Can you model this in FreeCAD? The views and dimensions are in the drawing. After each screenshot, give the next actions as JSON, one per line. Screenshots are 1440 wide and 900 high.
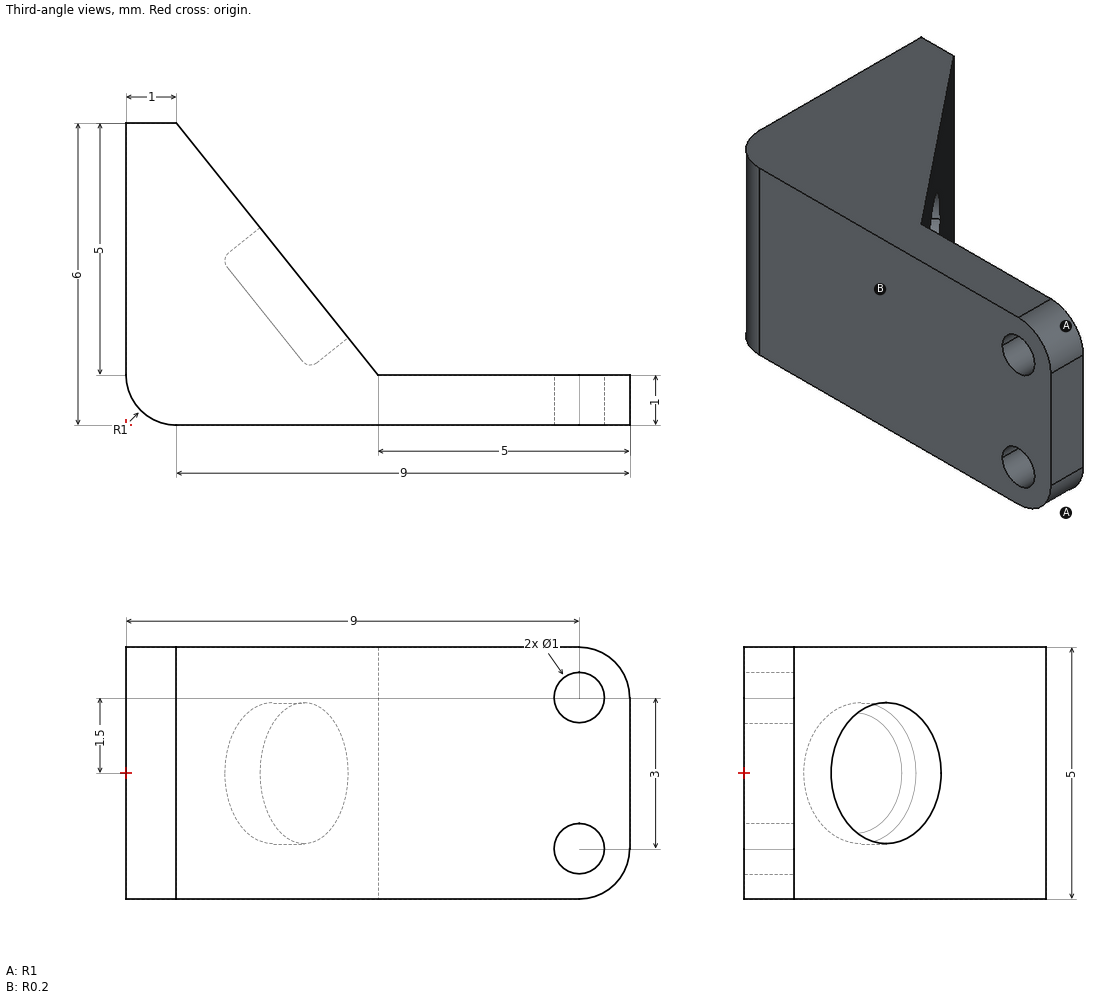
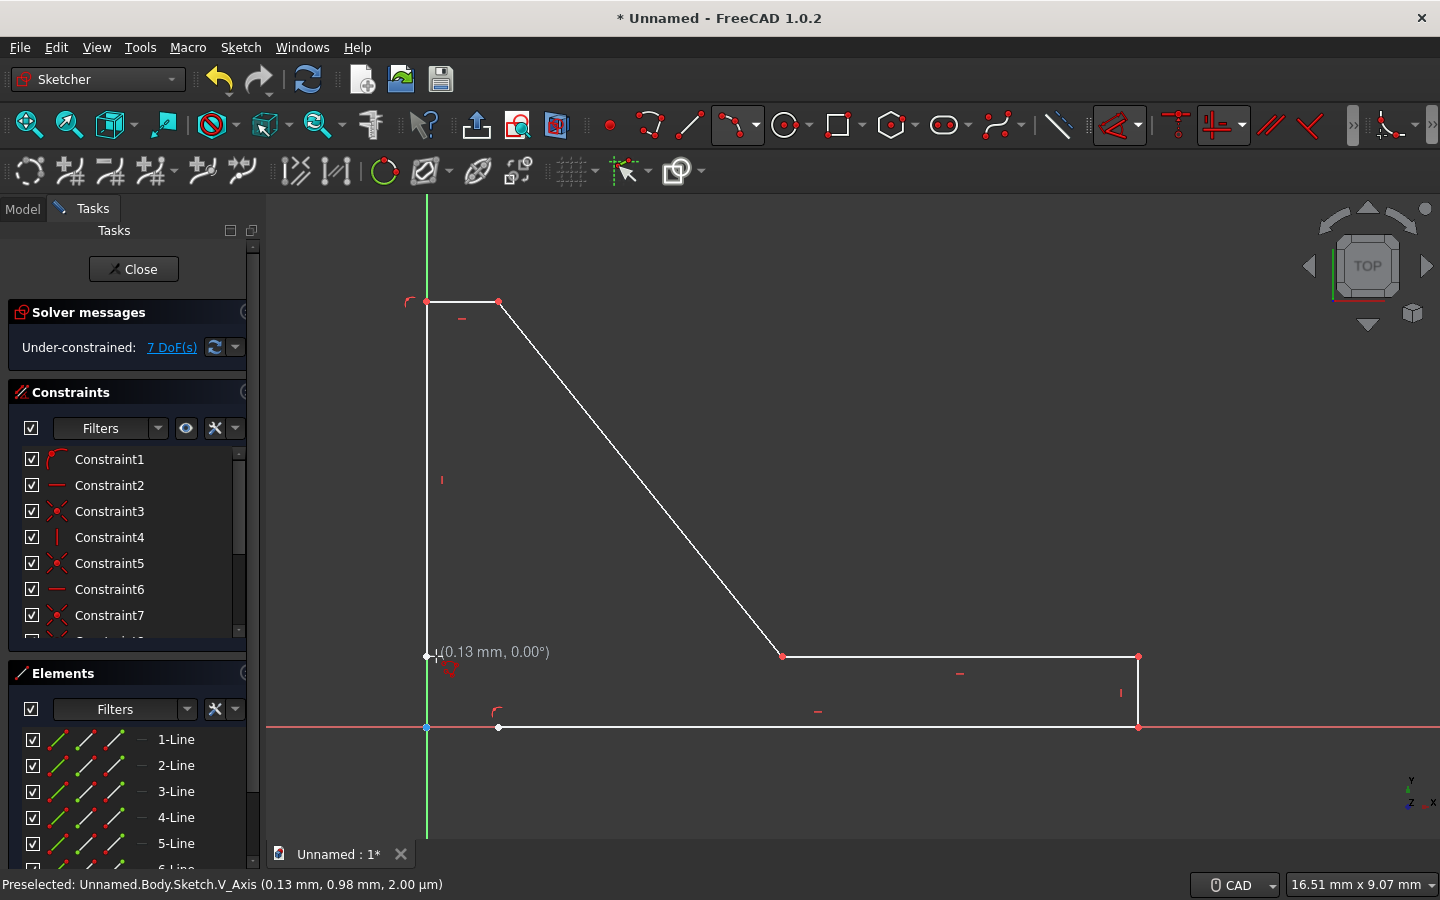
{"action": "left_click", "coordinate": [732, 126]}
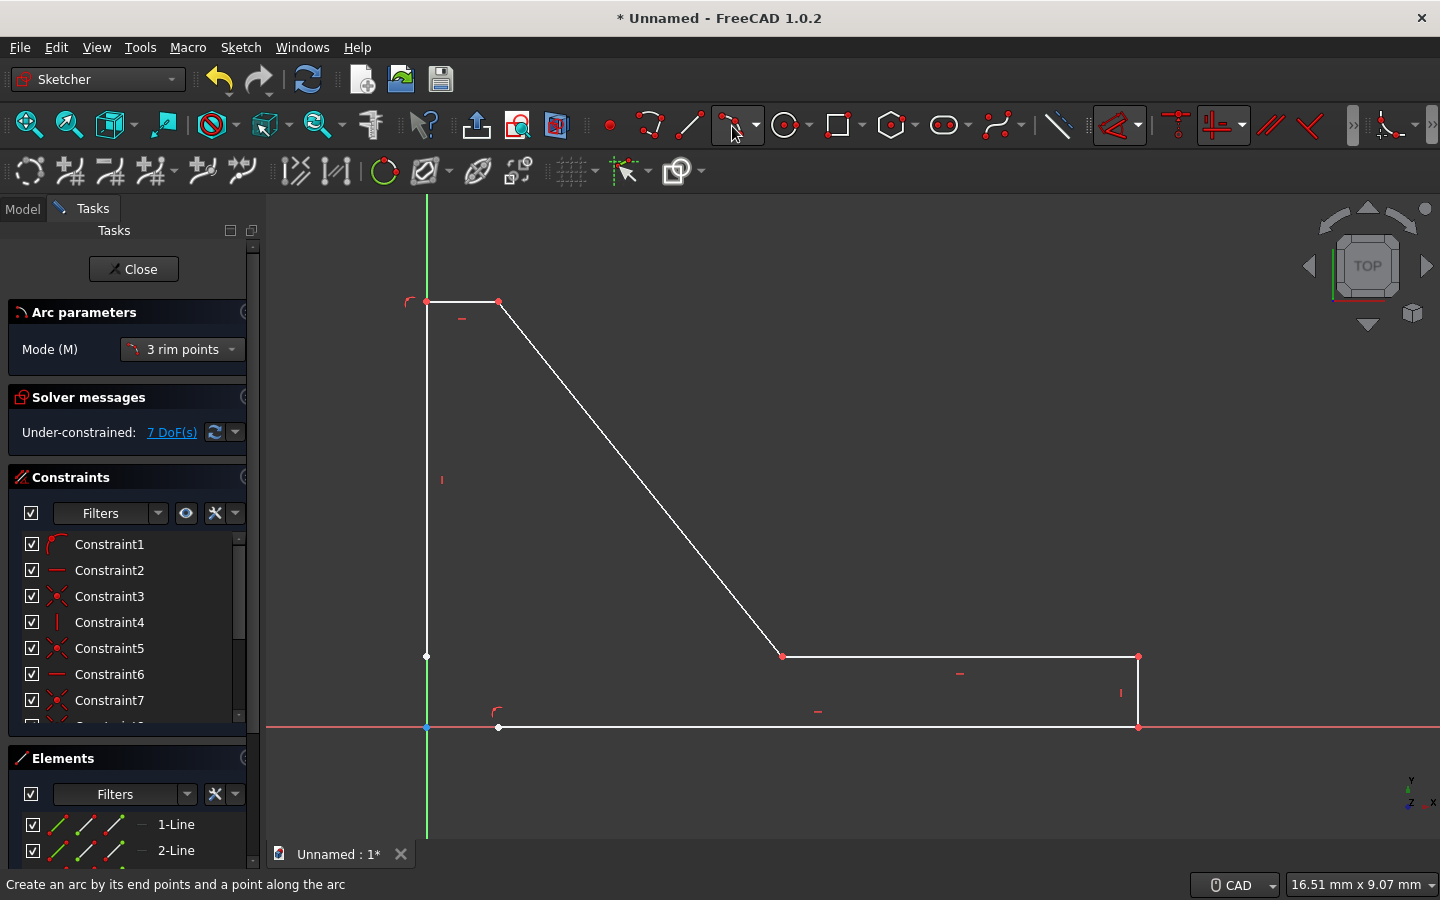
{"action": "left_click", "coordinate": [436, 656]}
{"action": "left_click", "coordinate": [498, 727]}
{"action": "left_click", "coordinate": [447, 706]}
{"action": "key", "text": "Escape"}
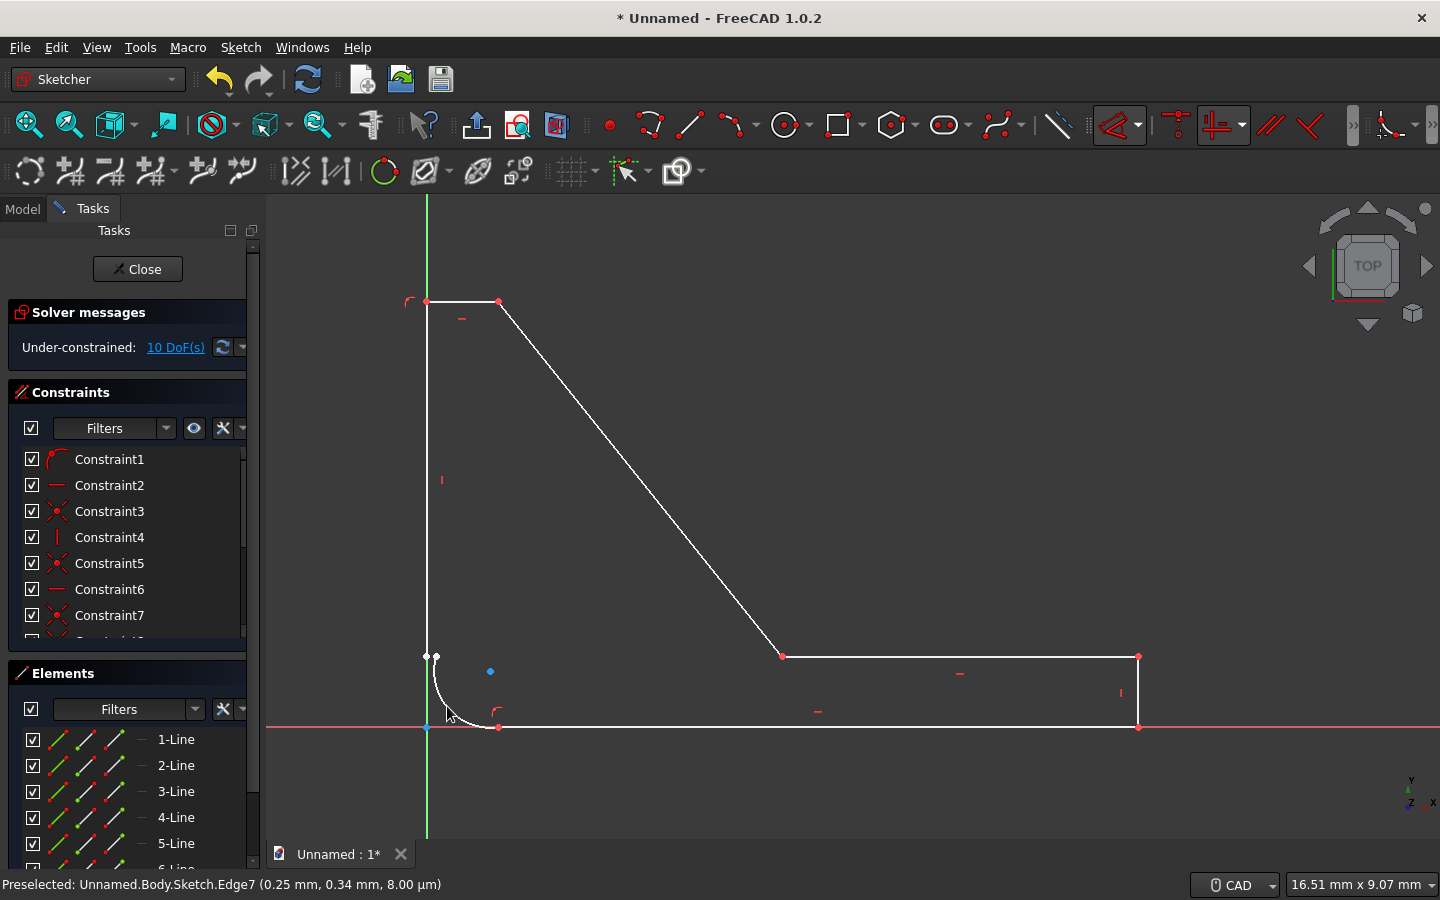
{"action": "left_click", "coordinate": [690, 727]}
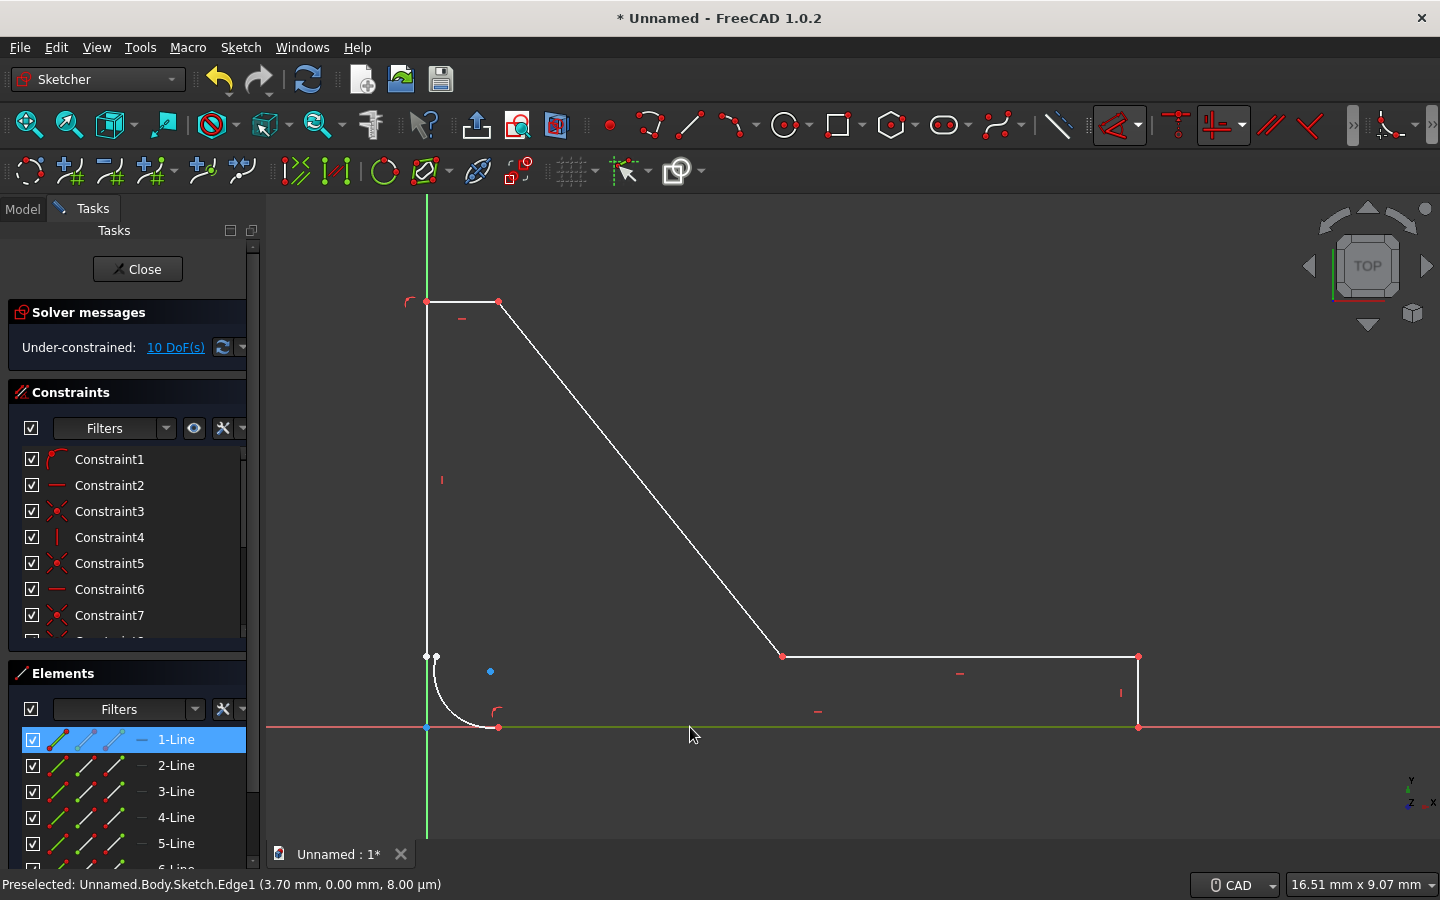
{"action": "scroll", "coordinate": [437, 690], "scroll_direction": "up", "scroll_amount": 2}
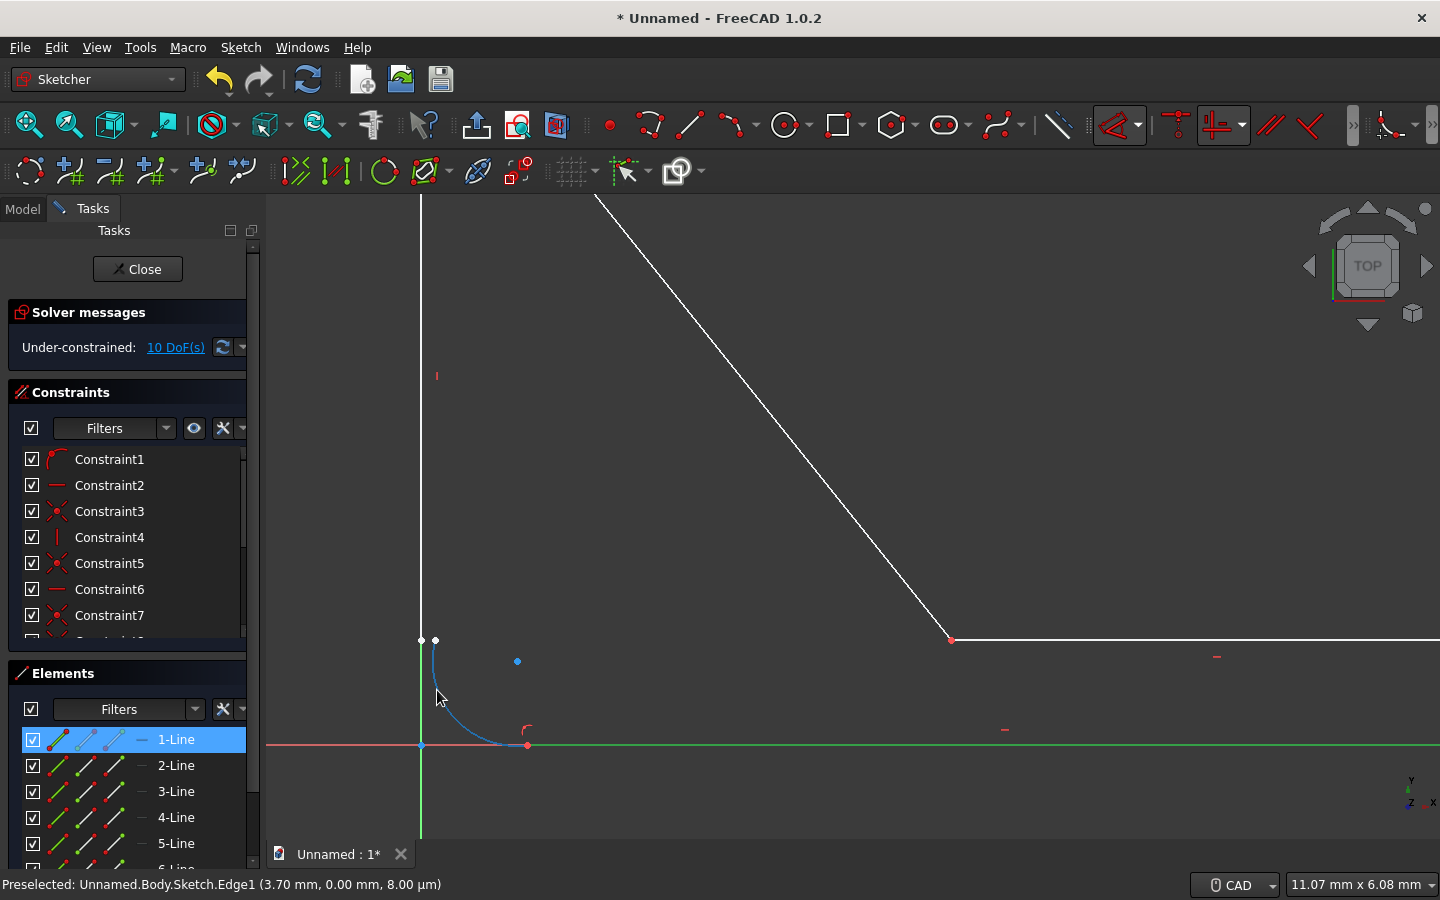
{"action": "left_click", "coordinate": [437, 689]}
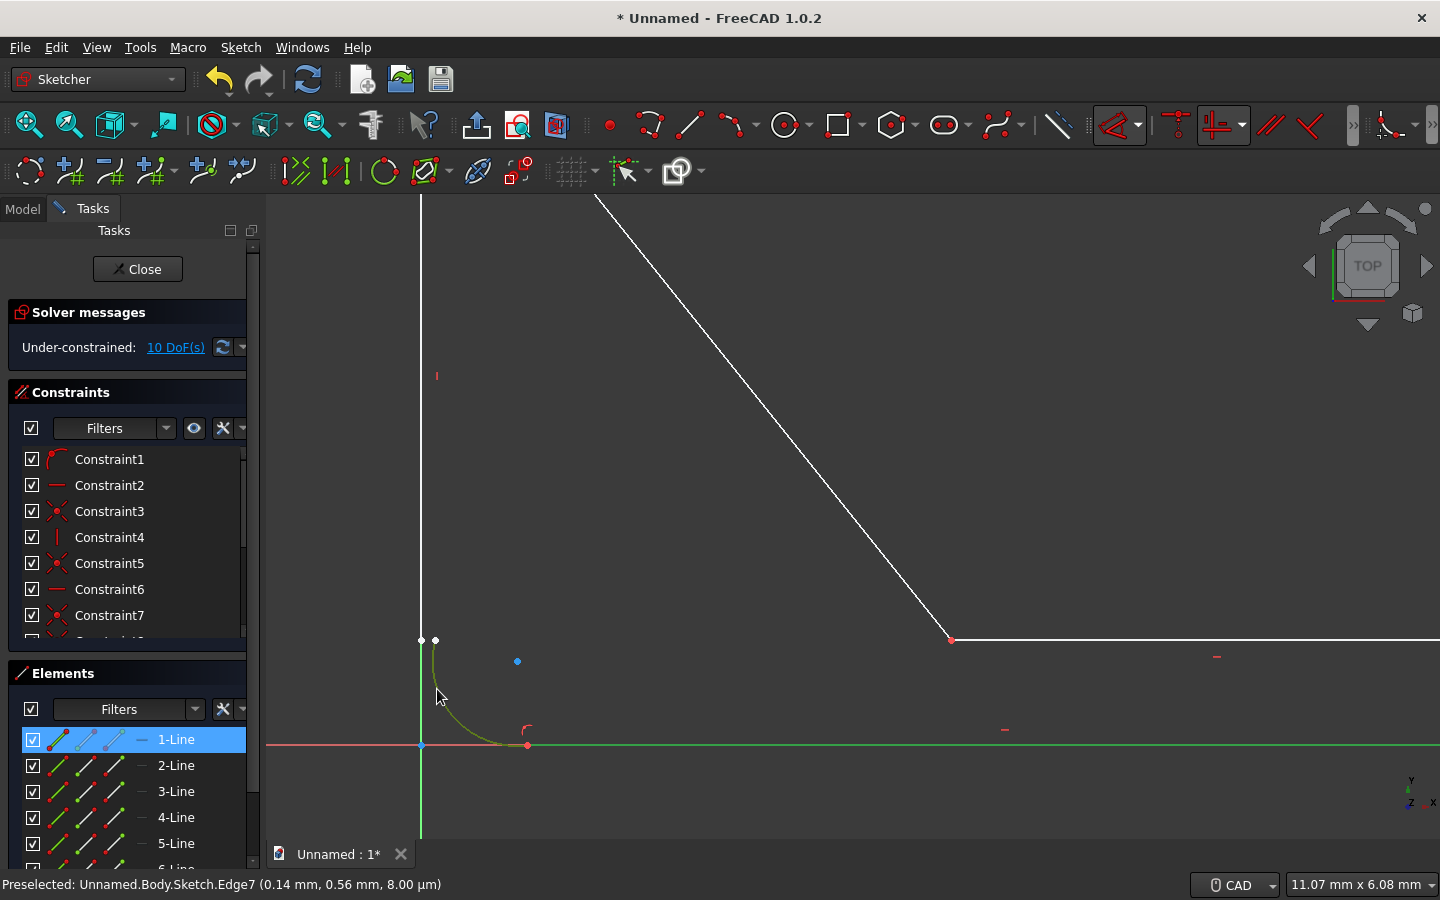
{"action": "key", "text": "t"}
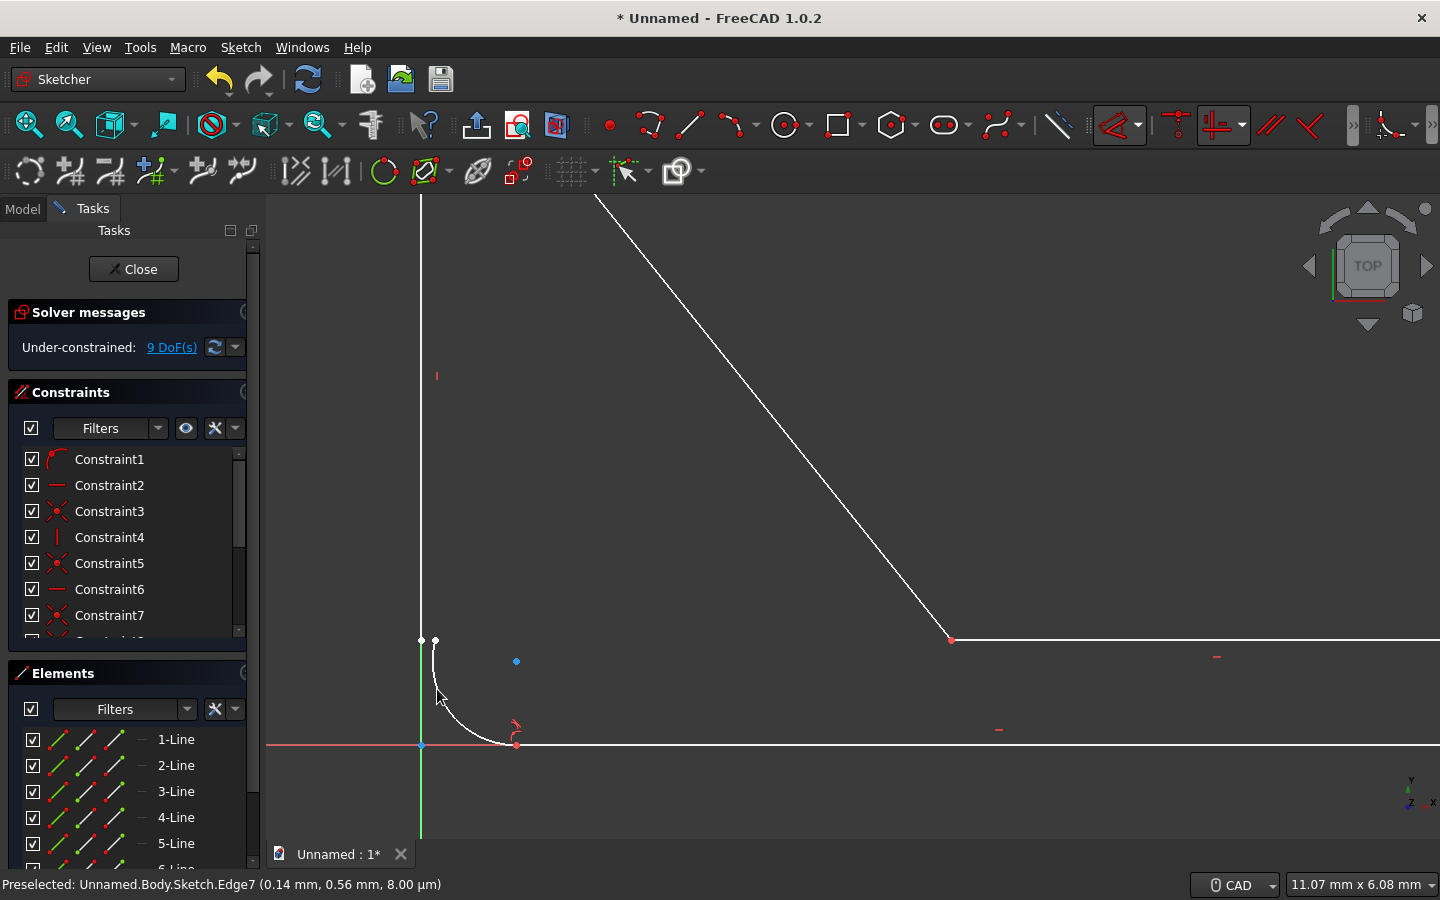
{"action": "left_click", "coordinate": [421, 270]}